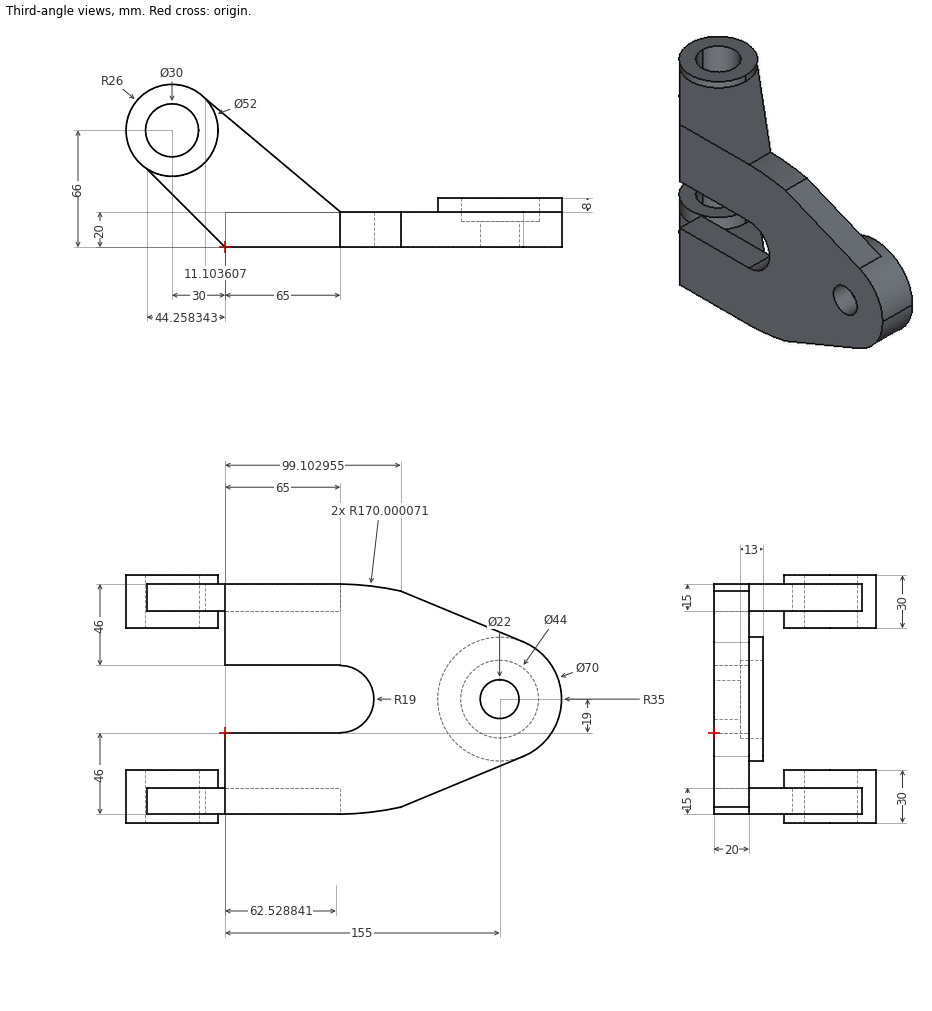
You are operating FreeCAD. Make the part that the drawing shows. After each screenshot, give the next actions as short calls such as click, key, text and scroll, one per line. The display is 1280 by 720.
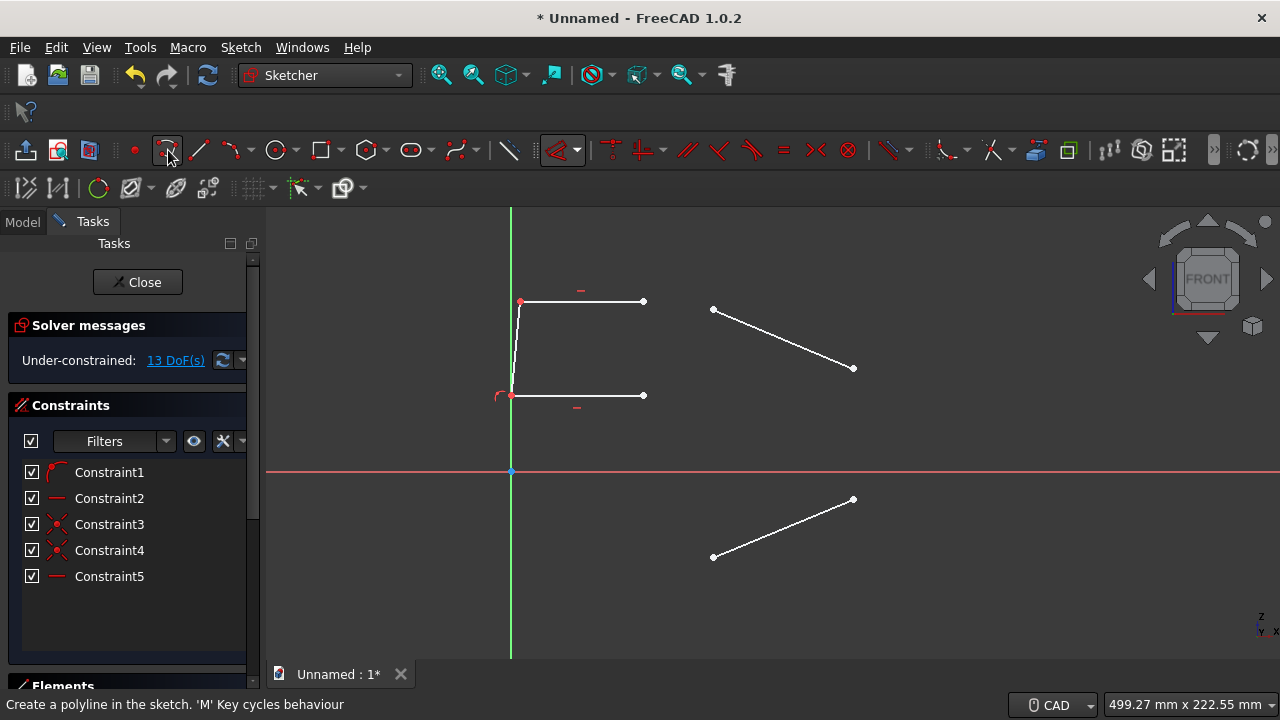
click(643, 565)
click(511, 565)
click(511, 472)
click(643, 463)
right_click(643, 463)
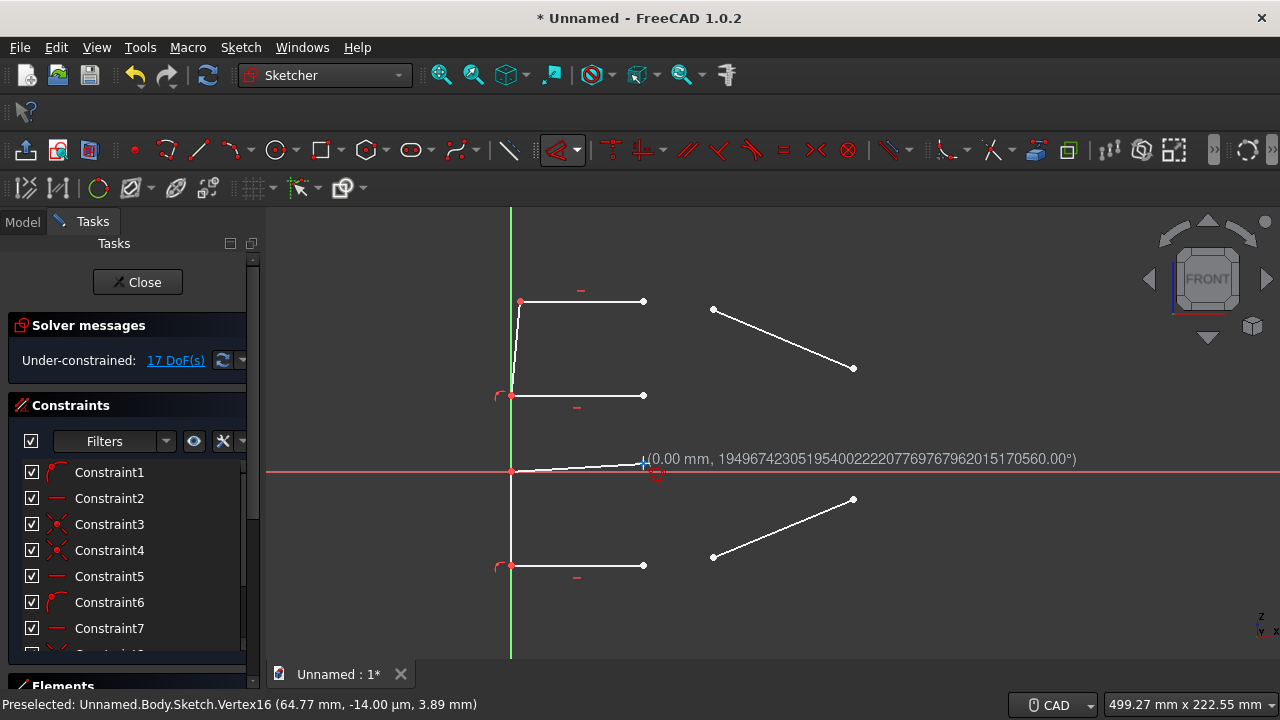
key(g)
key(3)
key(a)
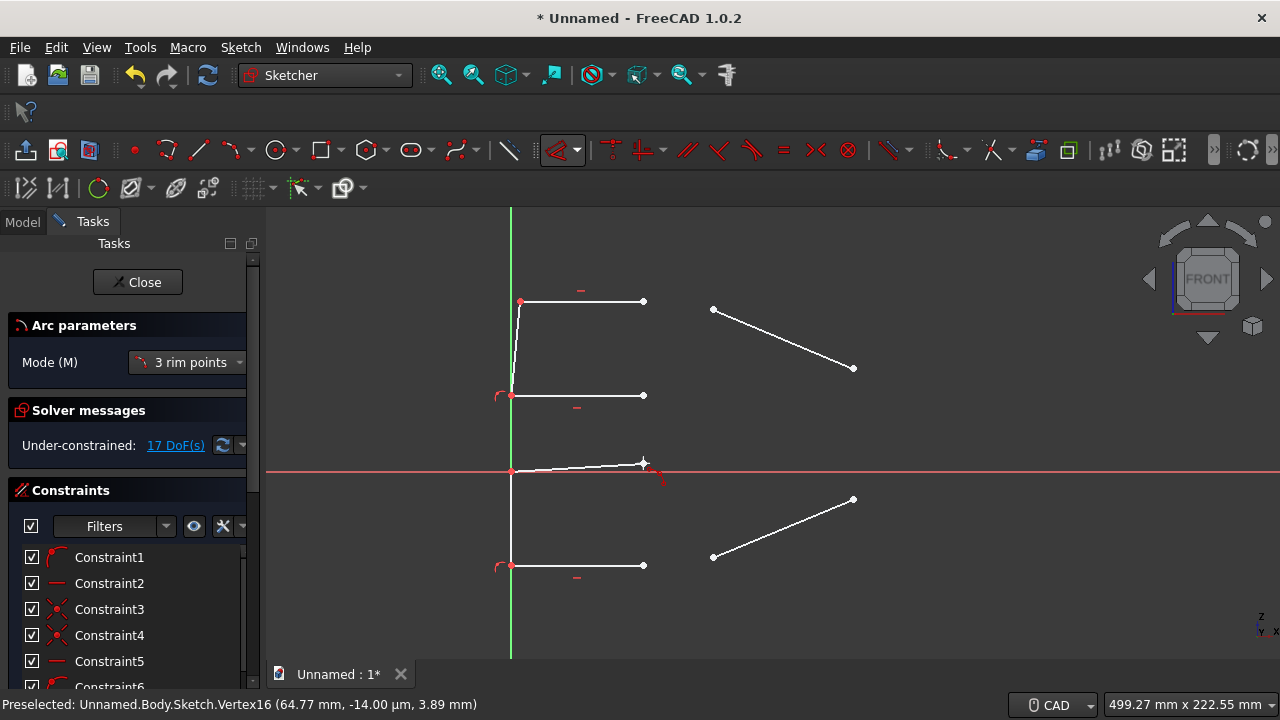
click(643, 302)
click(713, 310)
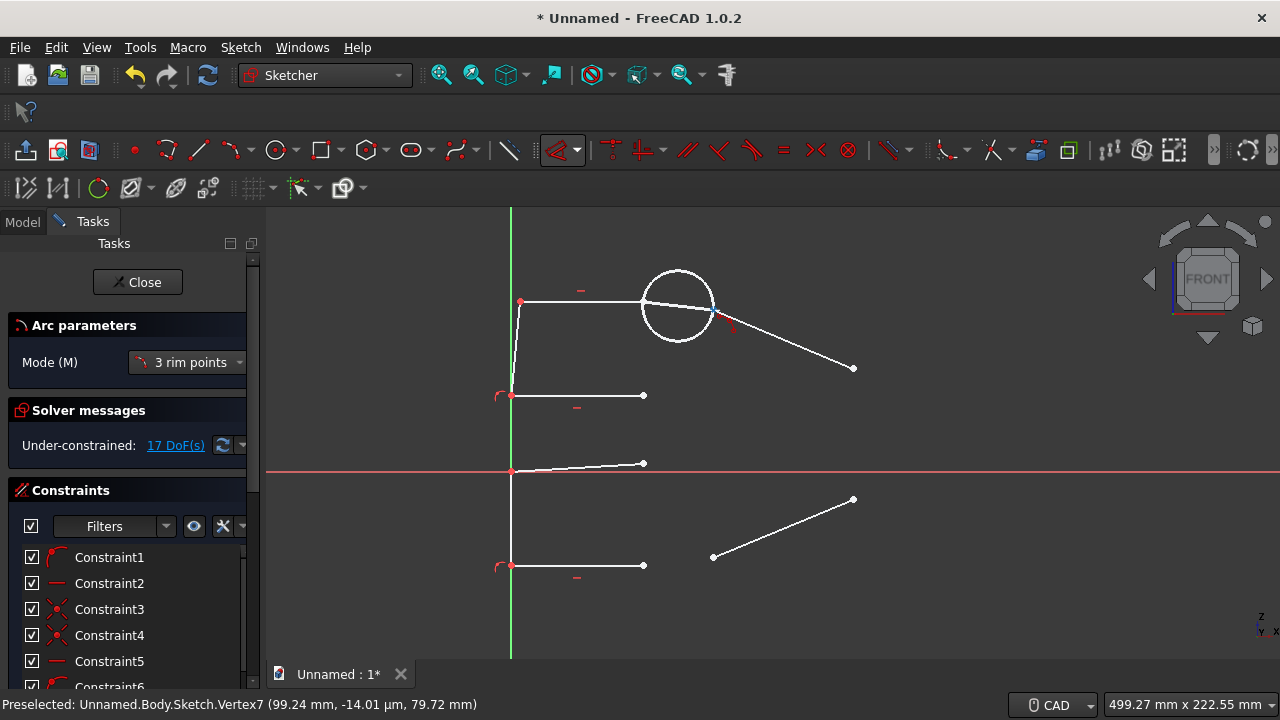
scroll(678, 304, up, 11)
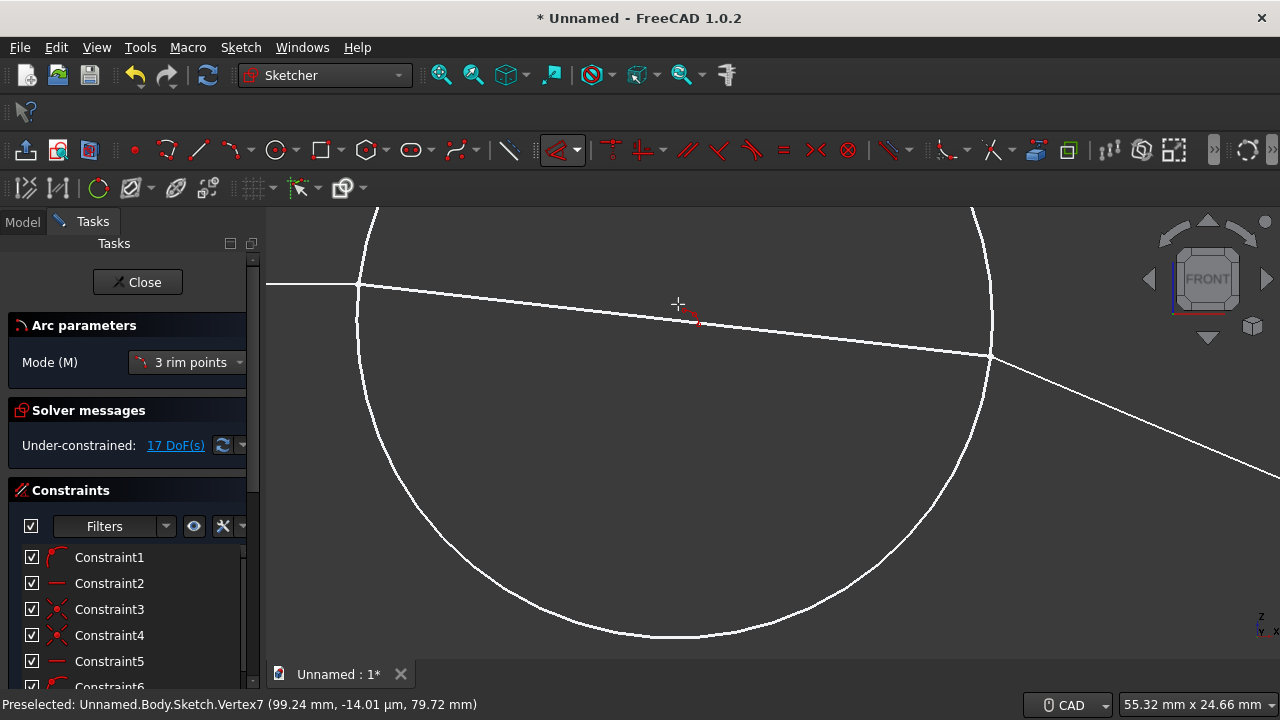
click(677, 298)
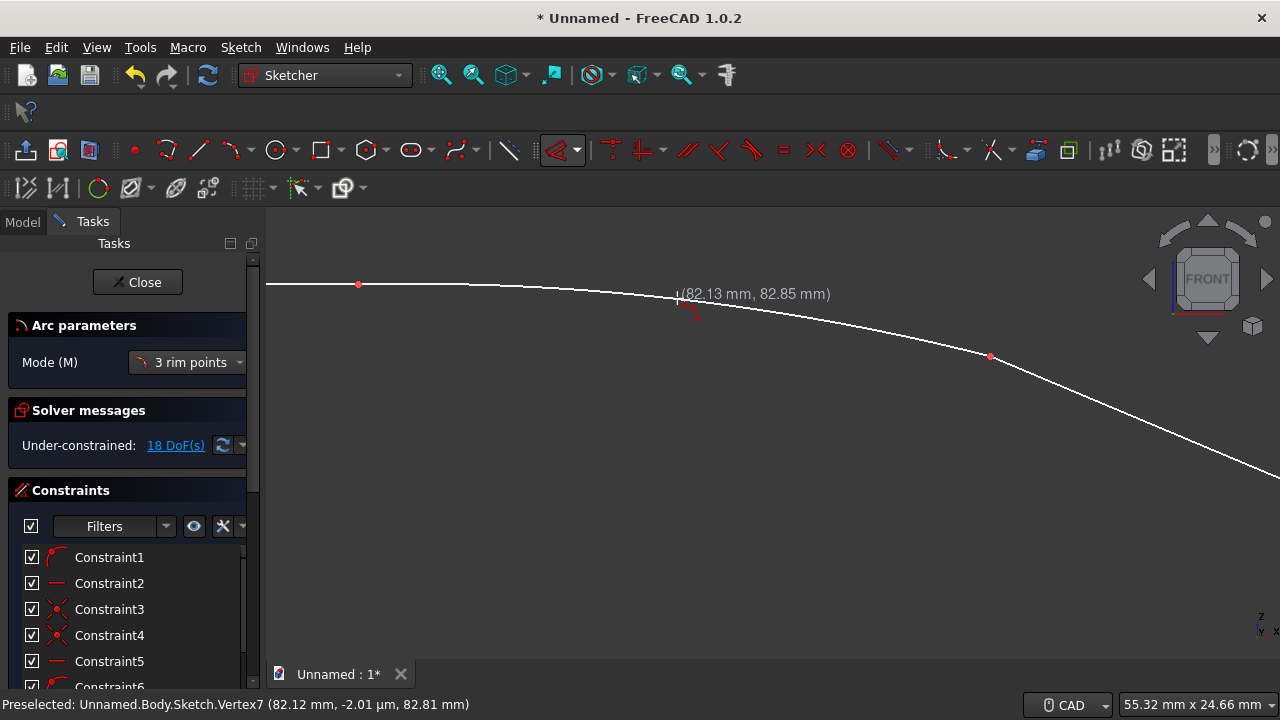
scroll(679, 304, down, 11)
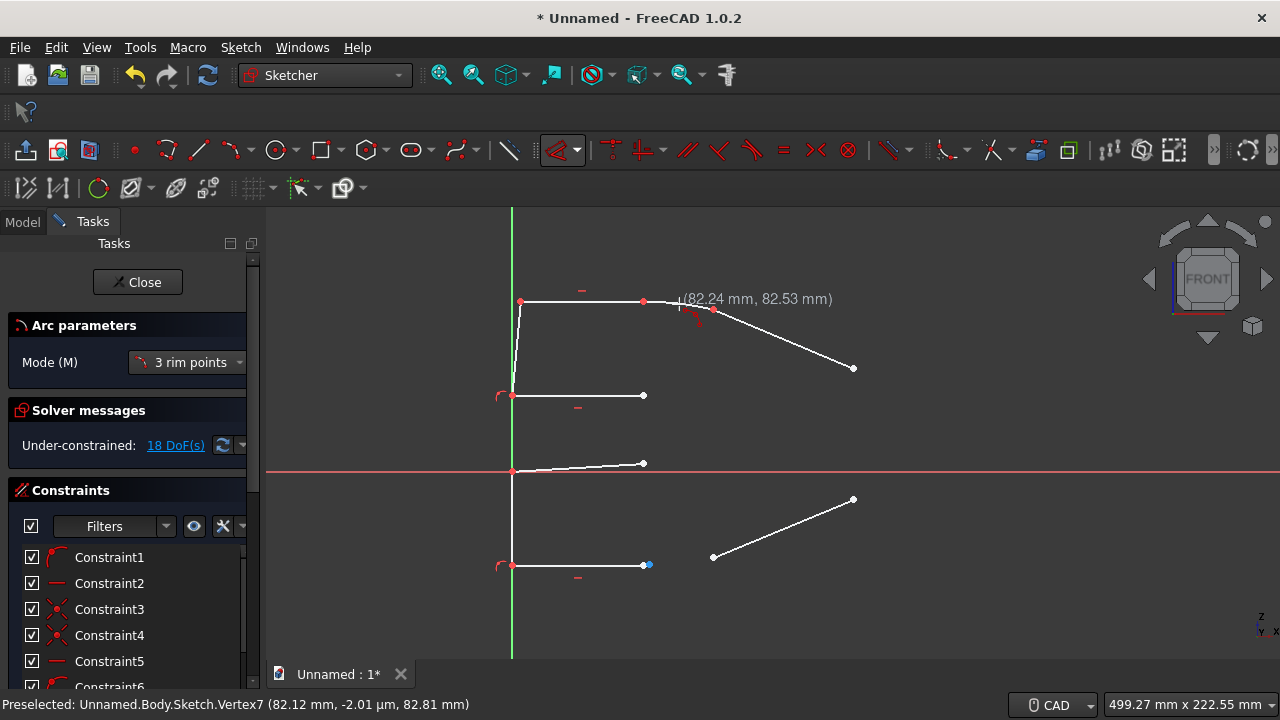
click(854, 369)
click(854, 500)
click(898, 433)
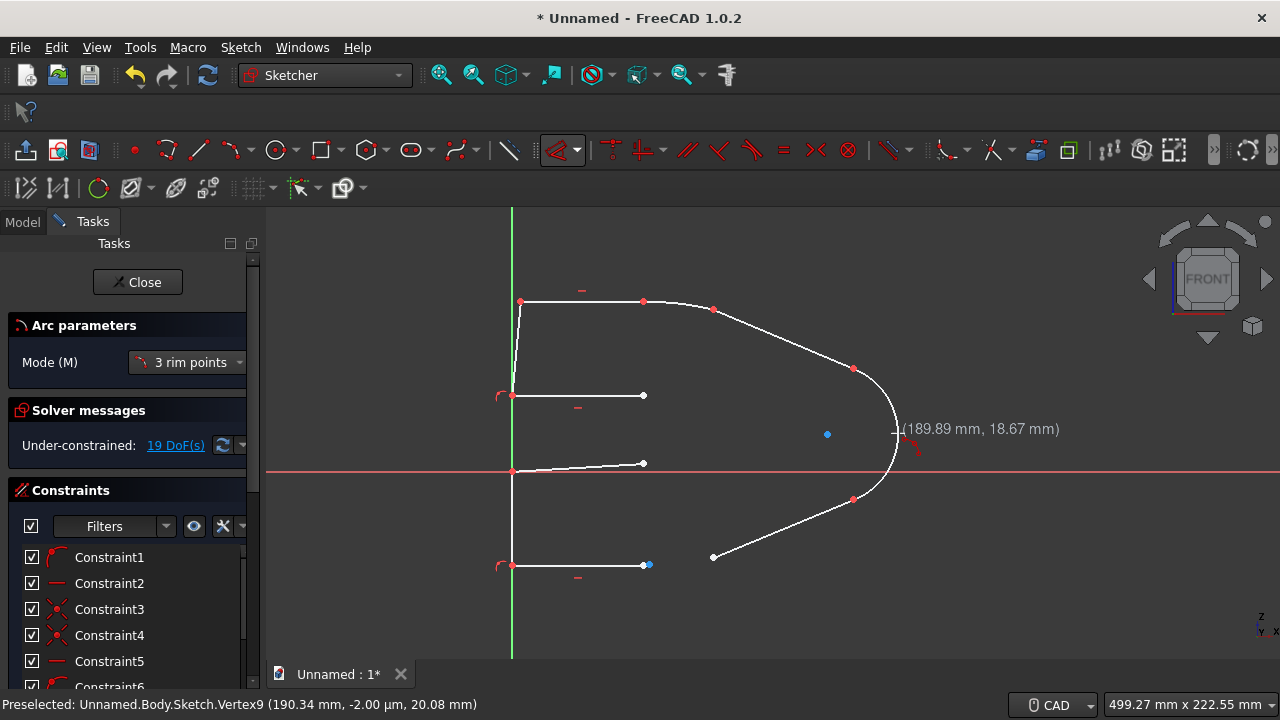
click(714, 558)
click(644, 566)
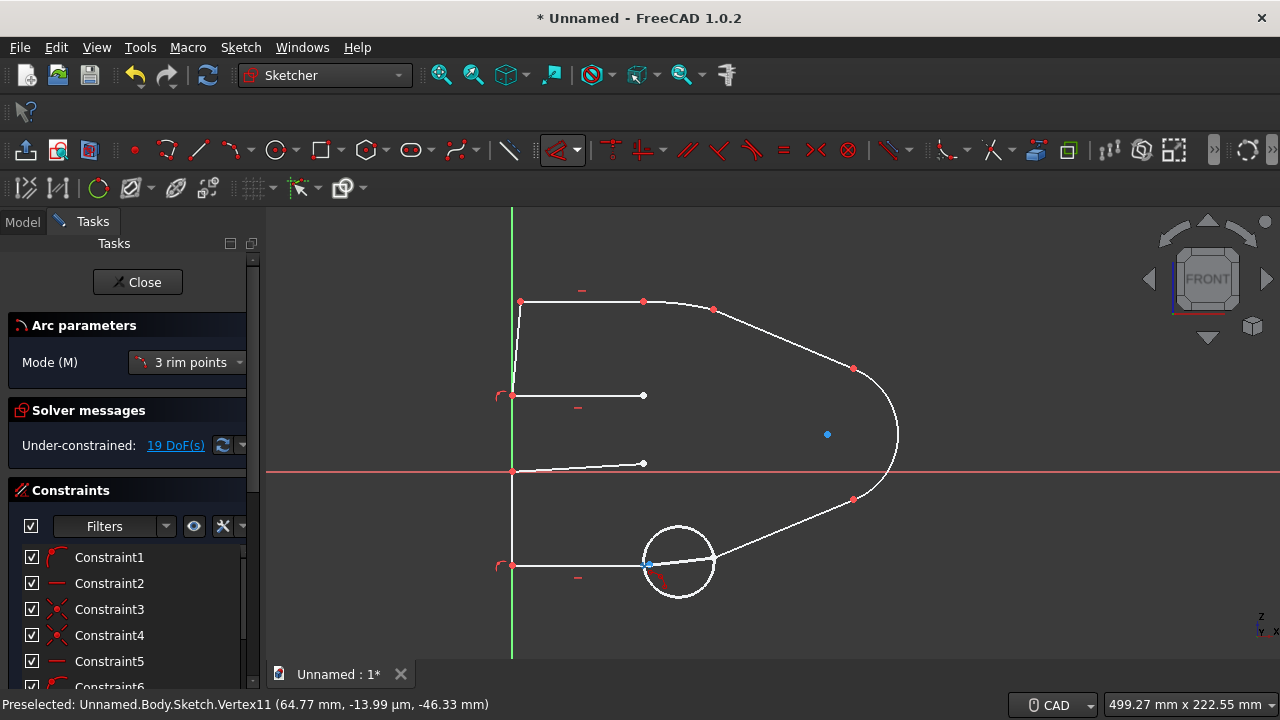
scroll(679, 563, up, 11)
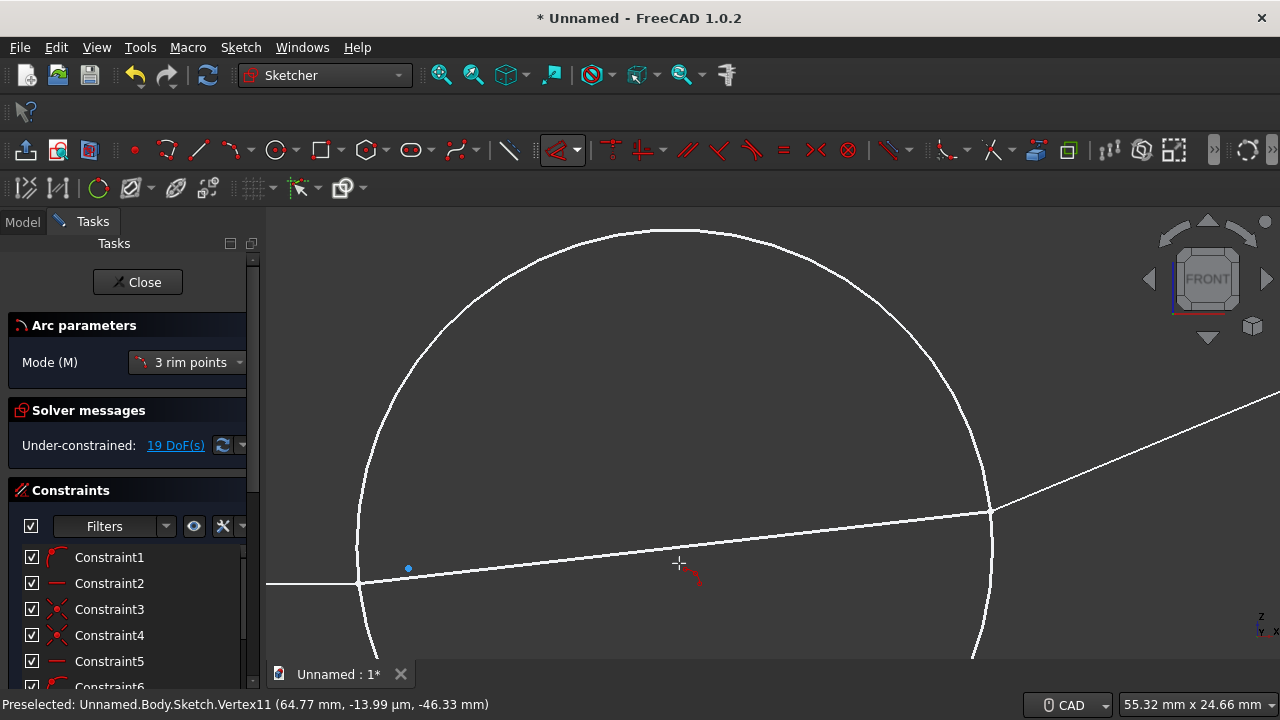
click(677, 557)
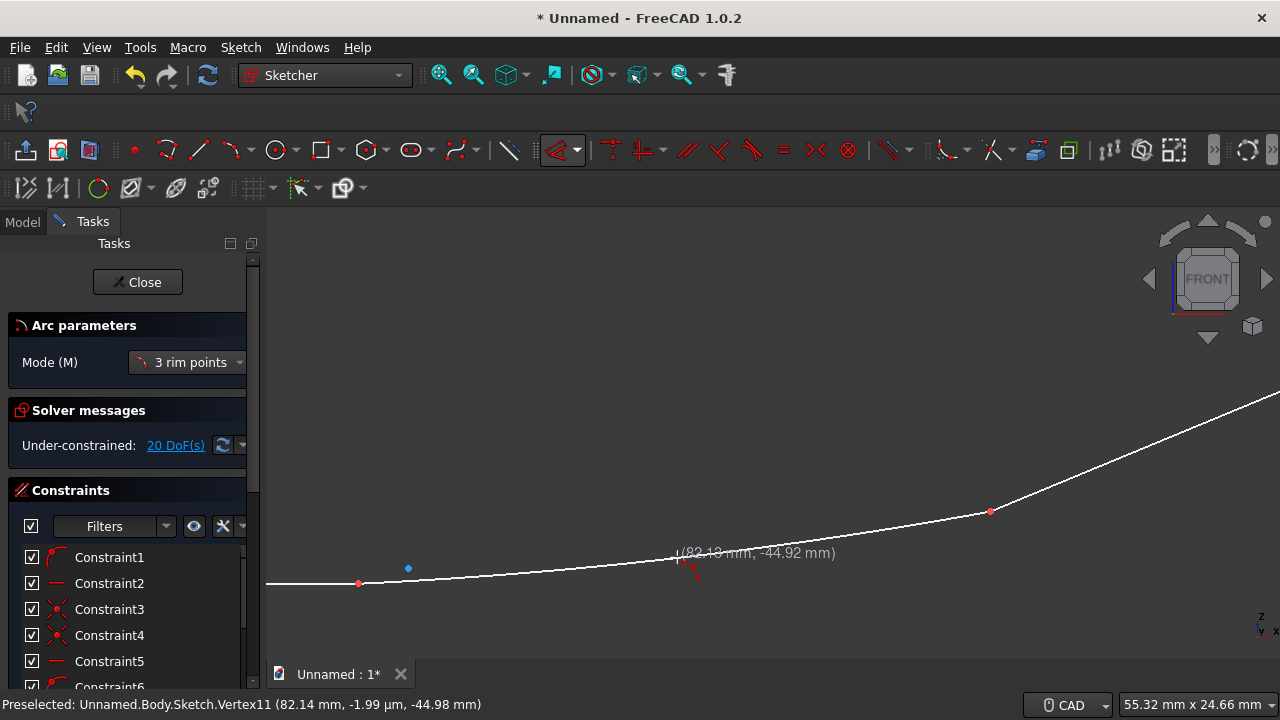
scroll(679, 563, down, 11)